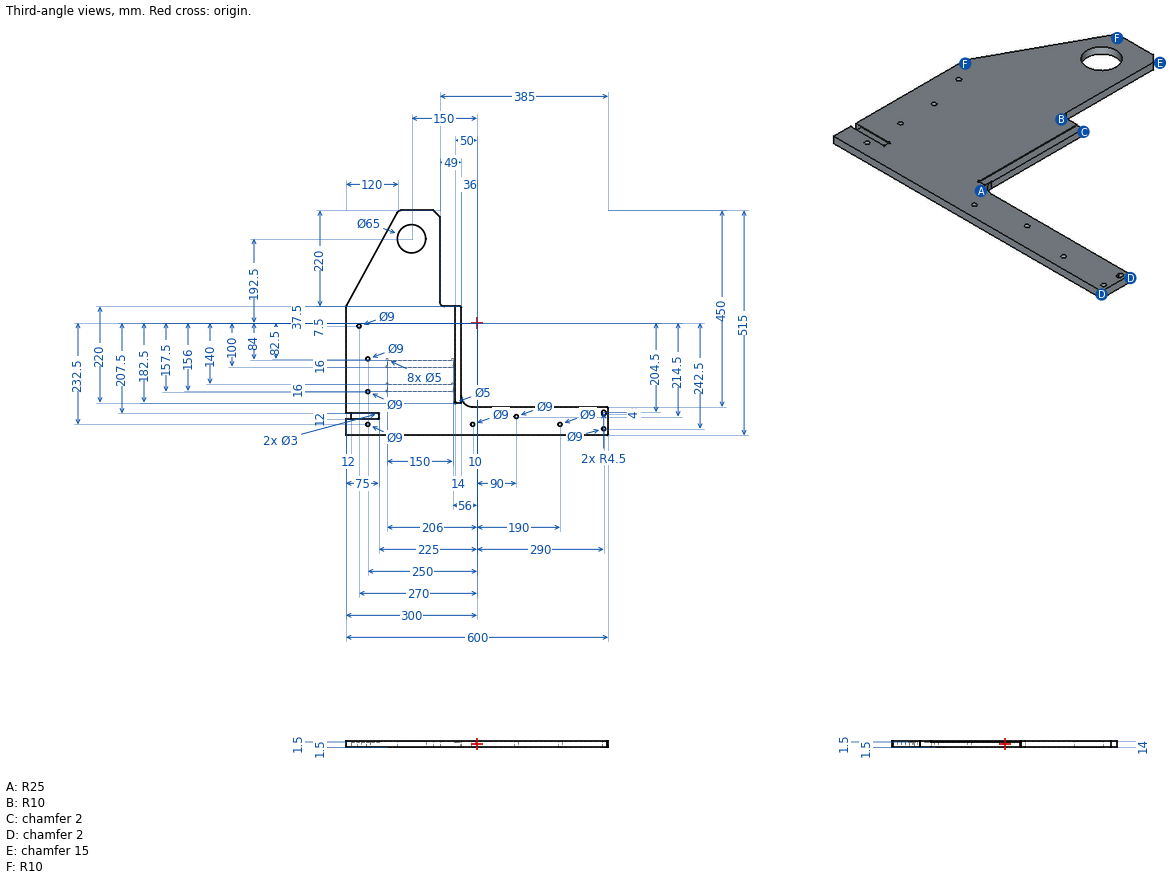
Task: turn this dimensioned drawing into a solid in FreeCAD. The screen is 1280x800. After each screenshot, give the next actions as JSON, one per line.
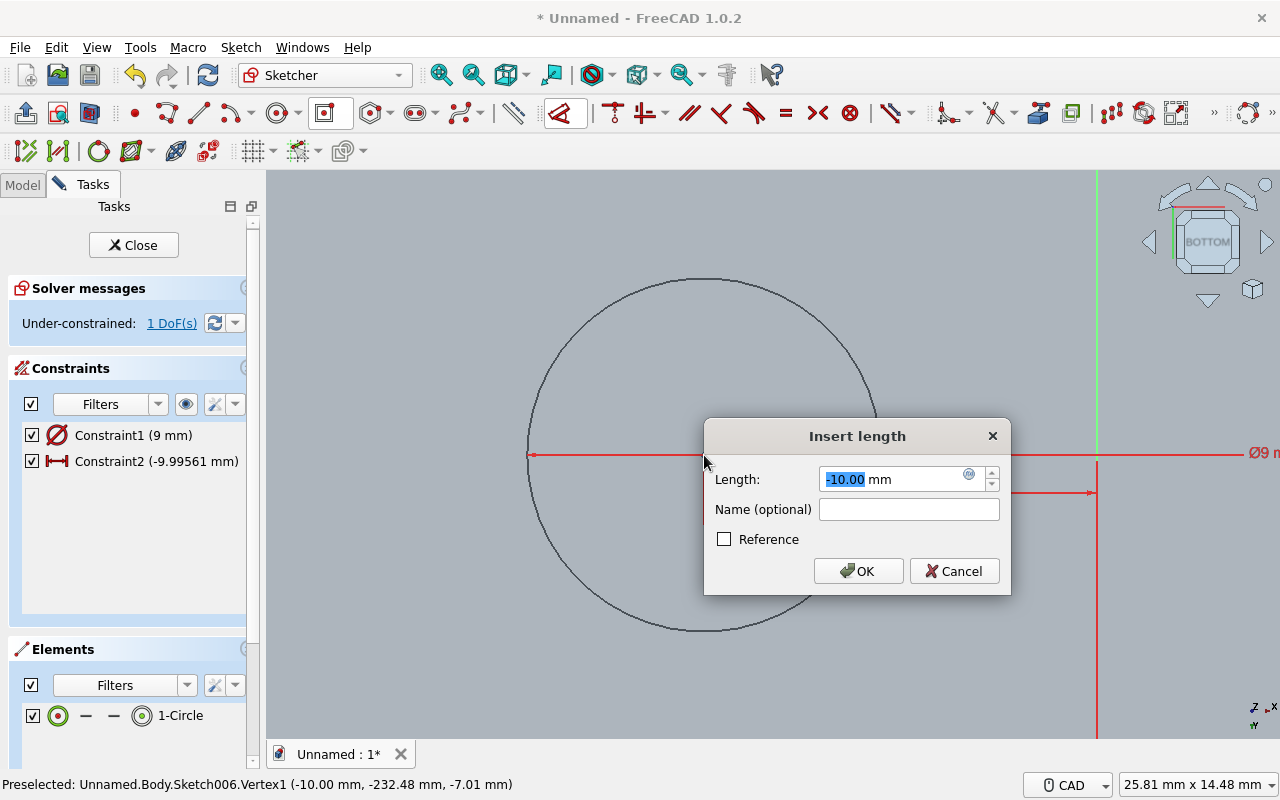
{"action": "type", "text": "-10"}
{"action": "key", "text": "Return"}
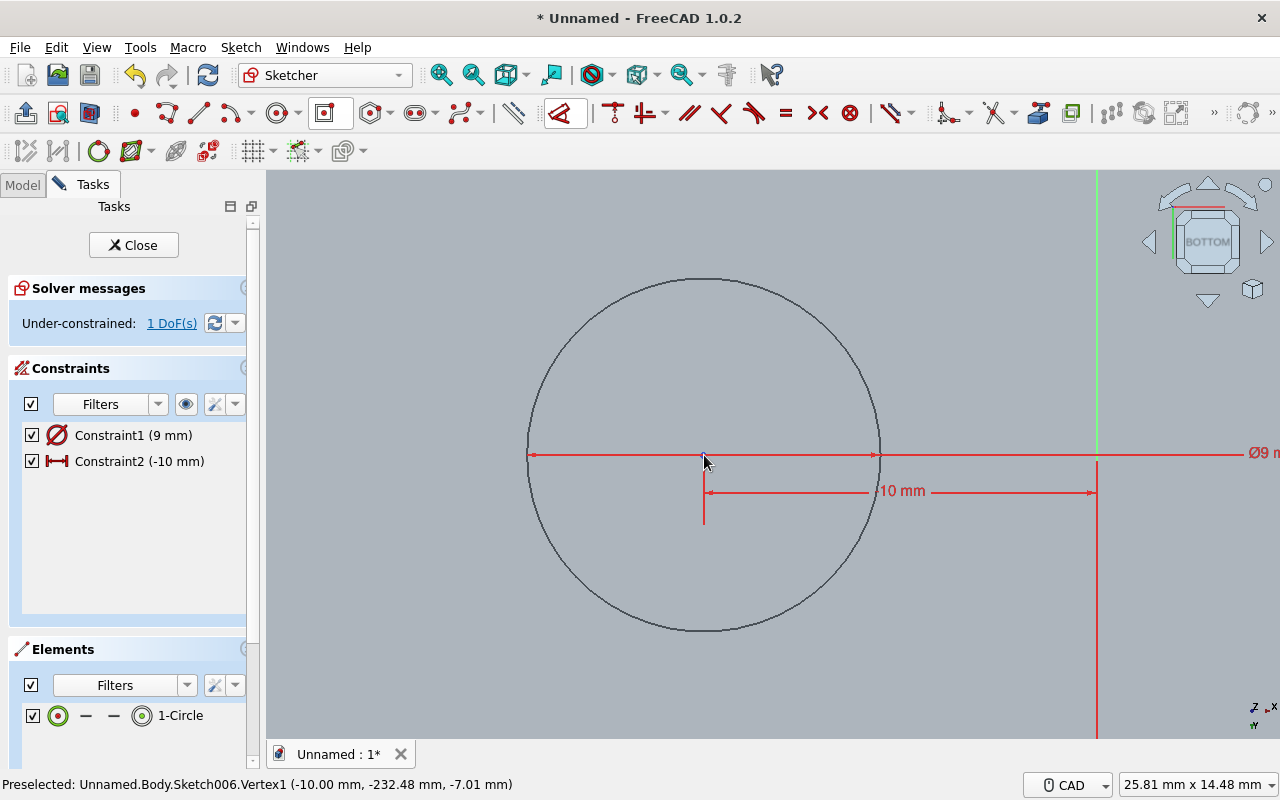
{"action": "left_click", "coordinate": [704, 455]}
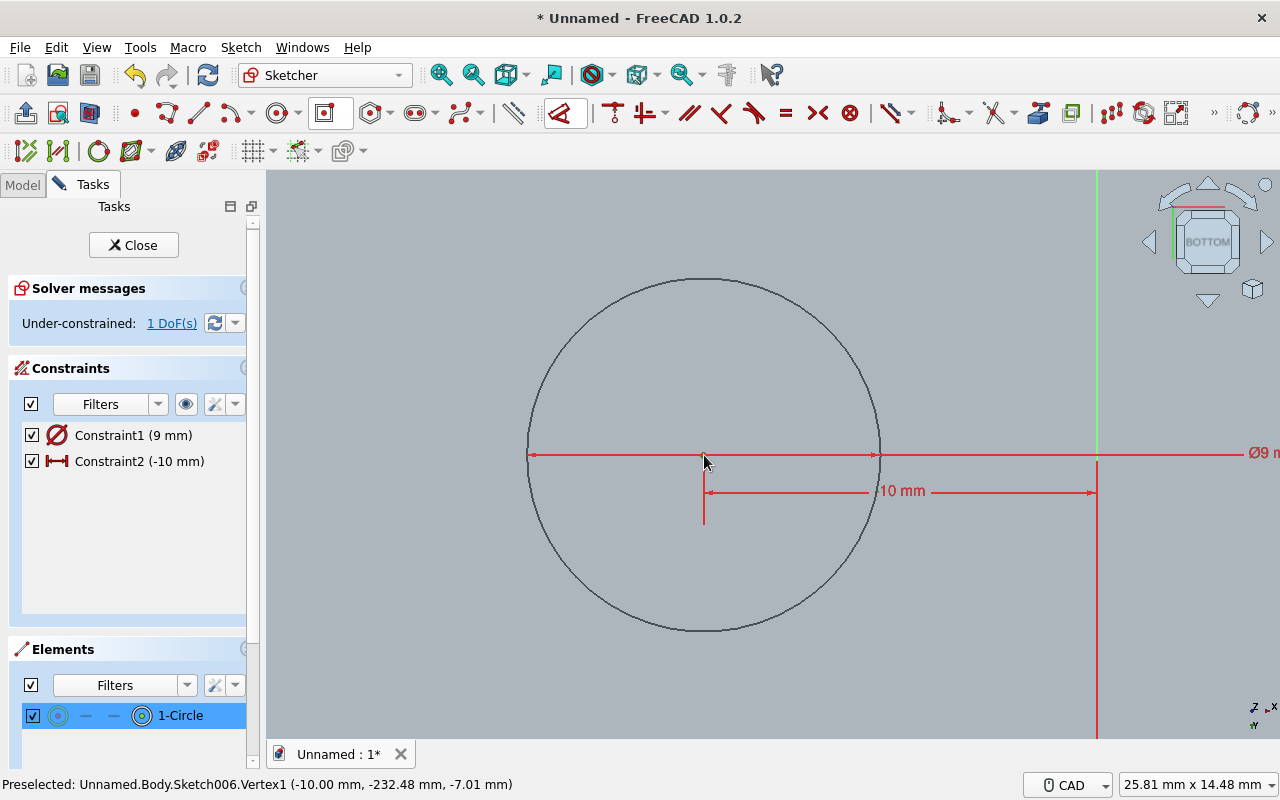
{"action": "left_click", "coordinate": [582, 114]}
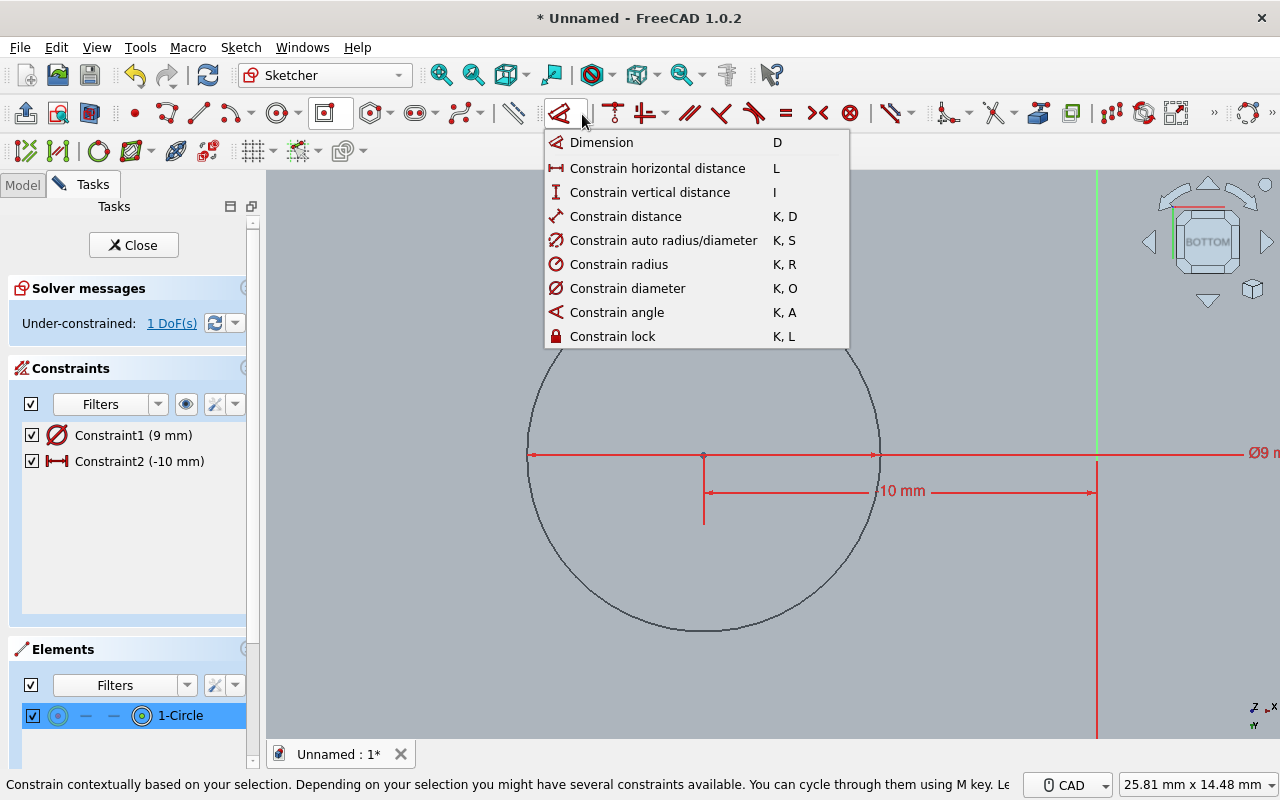
{"action": "left_click", "coordinate": [697, 192]}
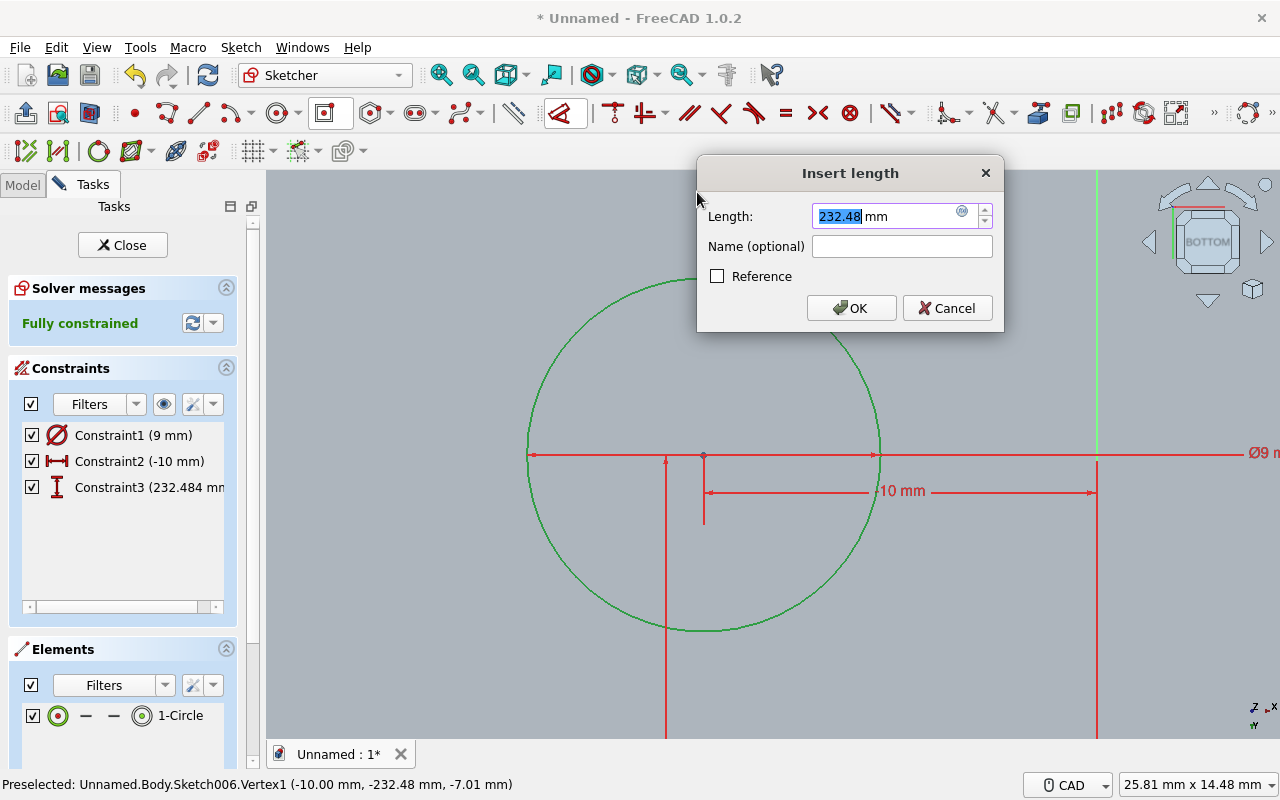
{"action": "type", "text": "232.5"}
{"action": "key", "text": "Return"}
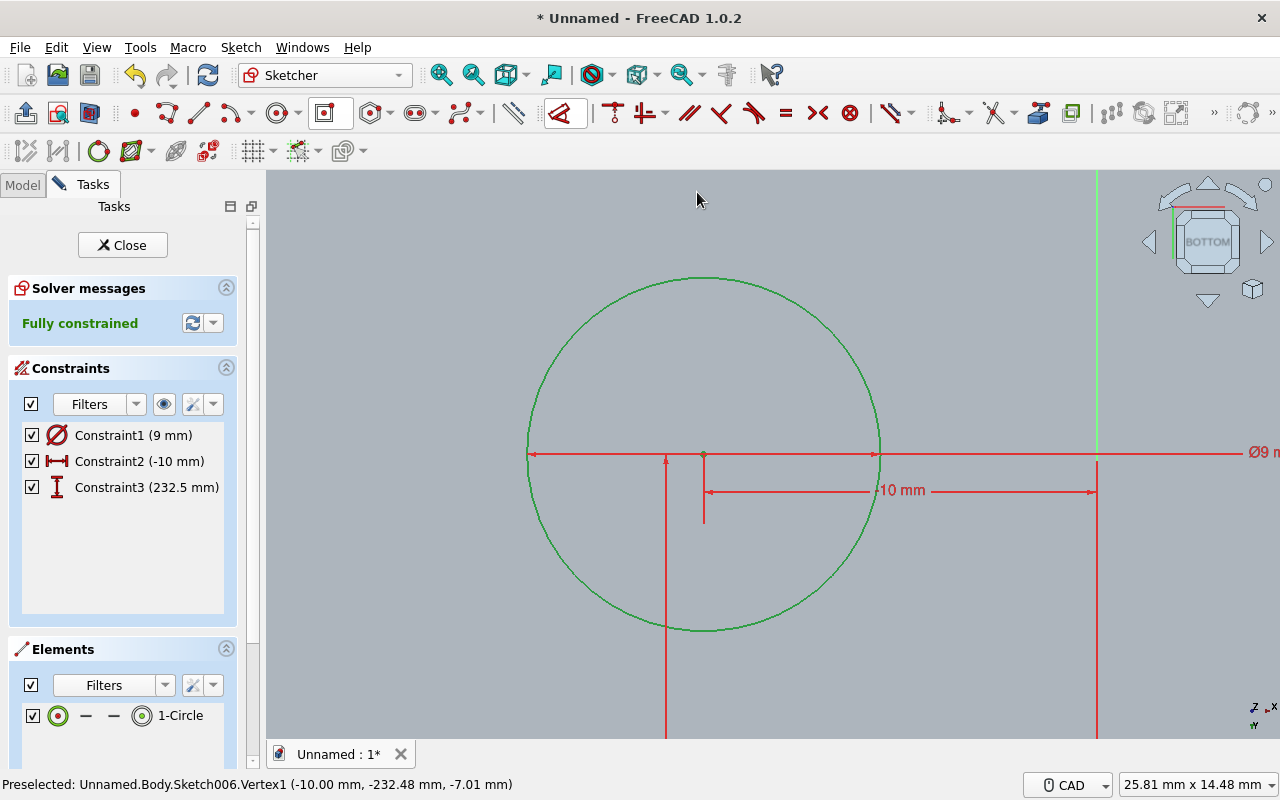
{"action": "left_click", "coordinate": [123, 245]}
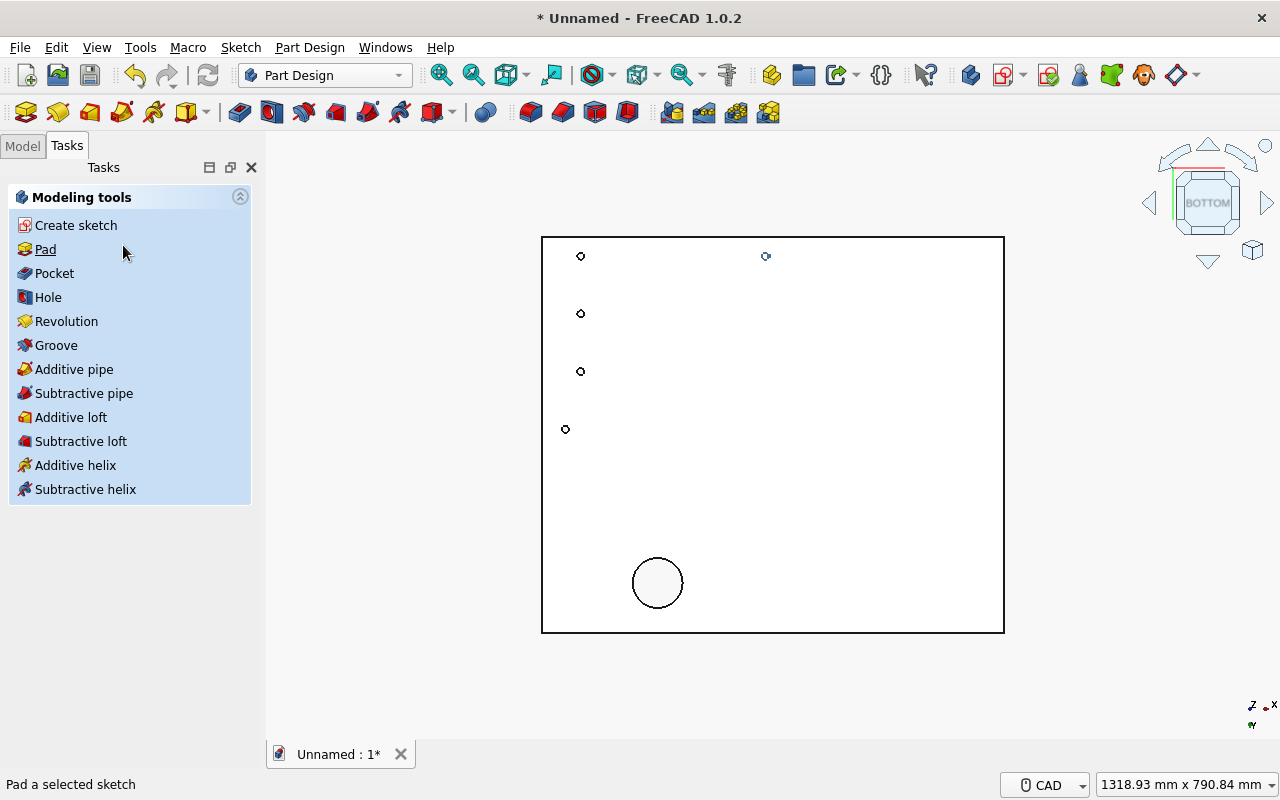
{"action": "left_click", "coordinate": [240, 112]}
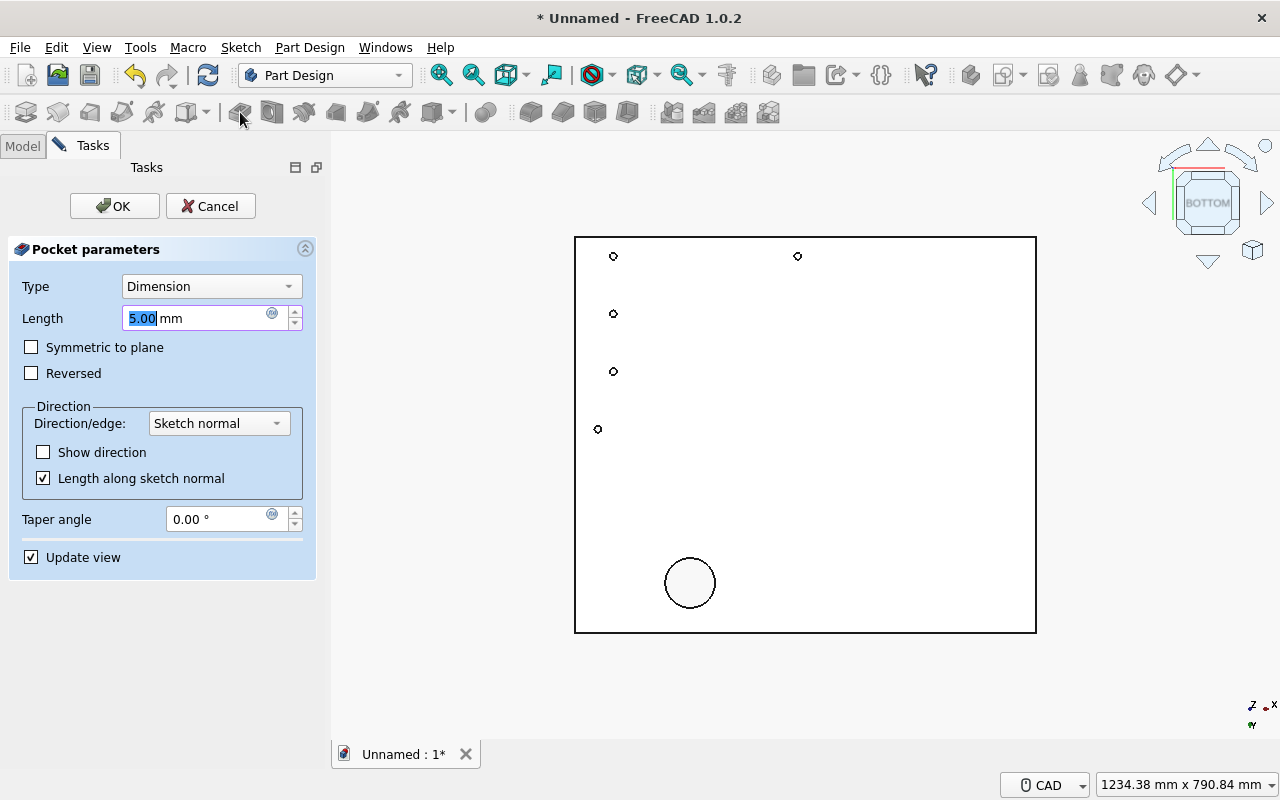
{"action": "left_click", "coordinate": [212, 286]}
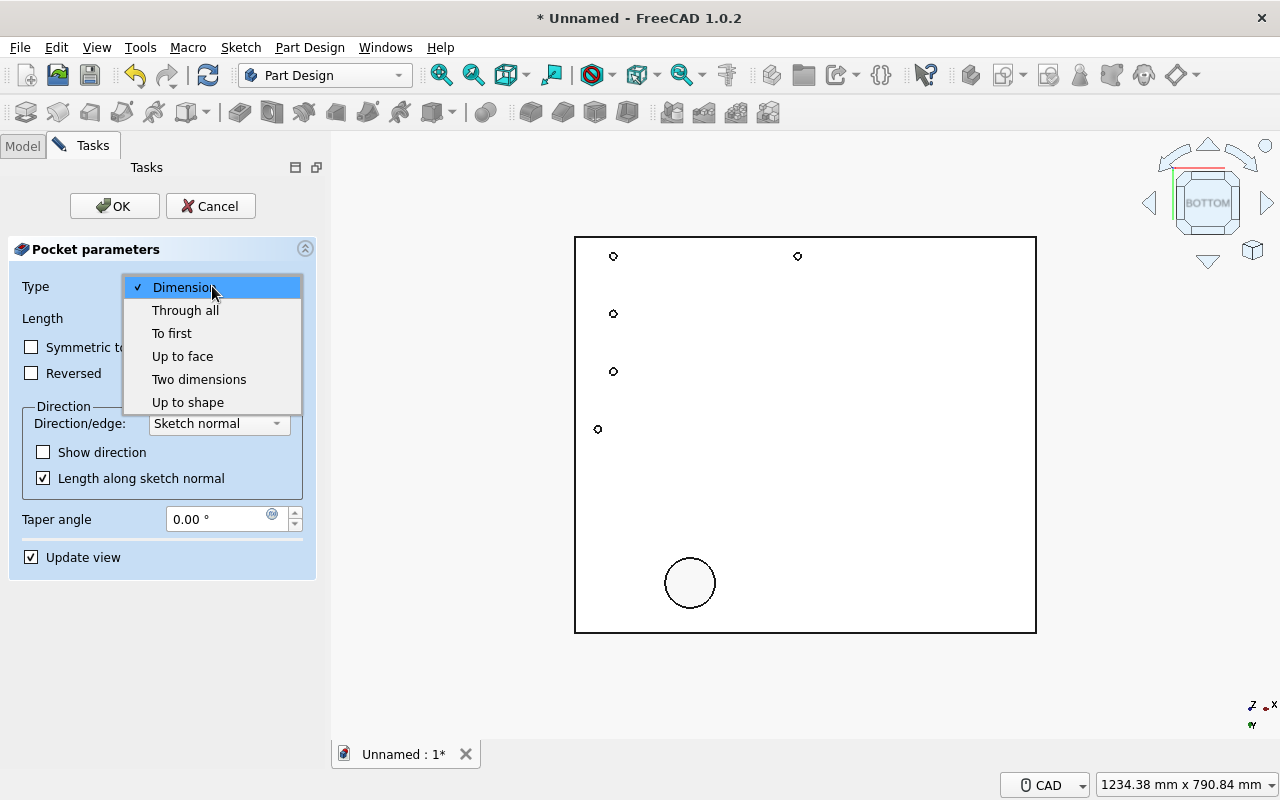
{"action": "left_click", "coordinate": [212, 334]}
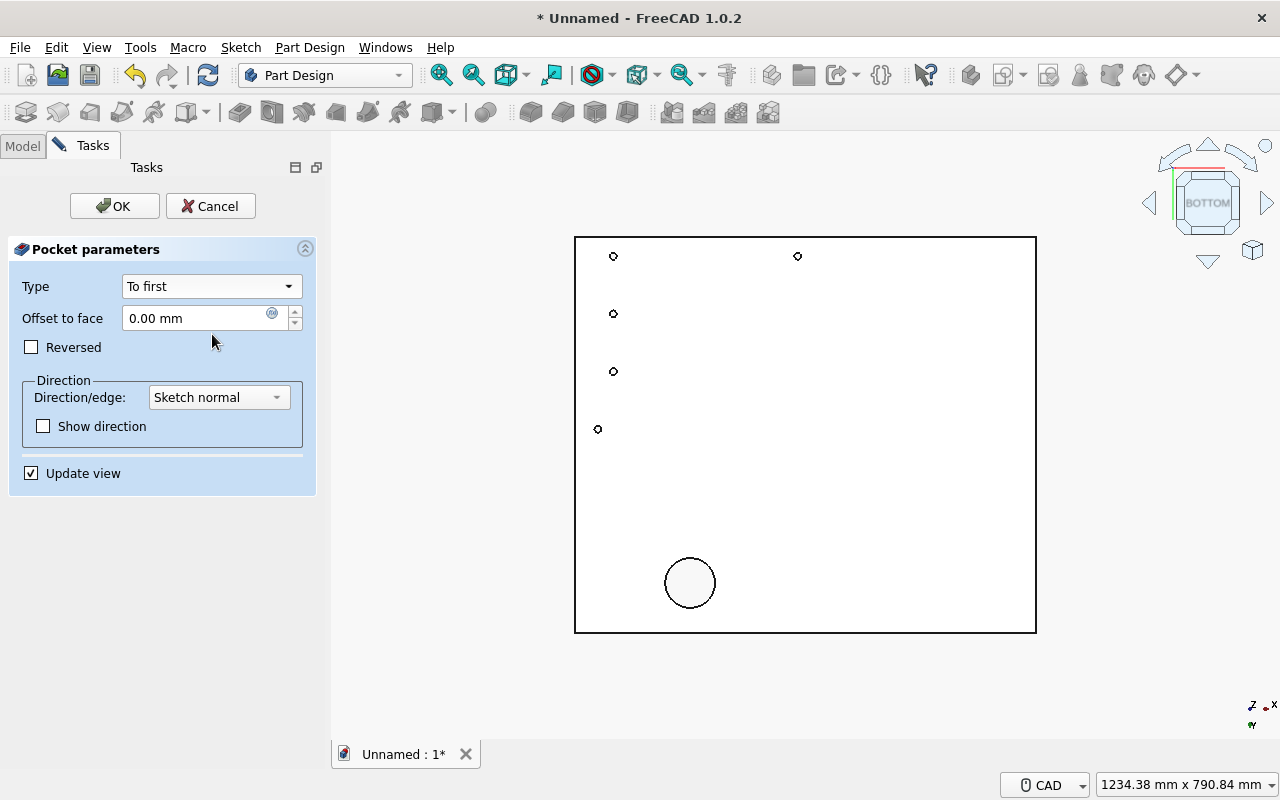
{"action": "left_click", "coordinate": [115, 206]}